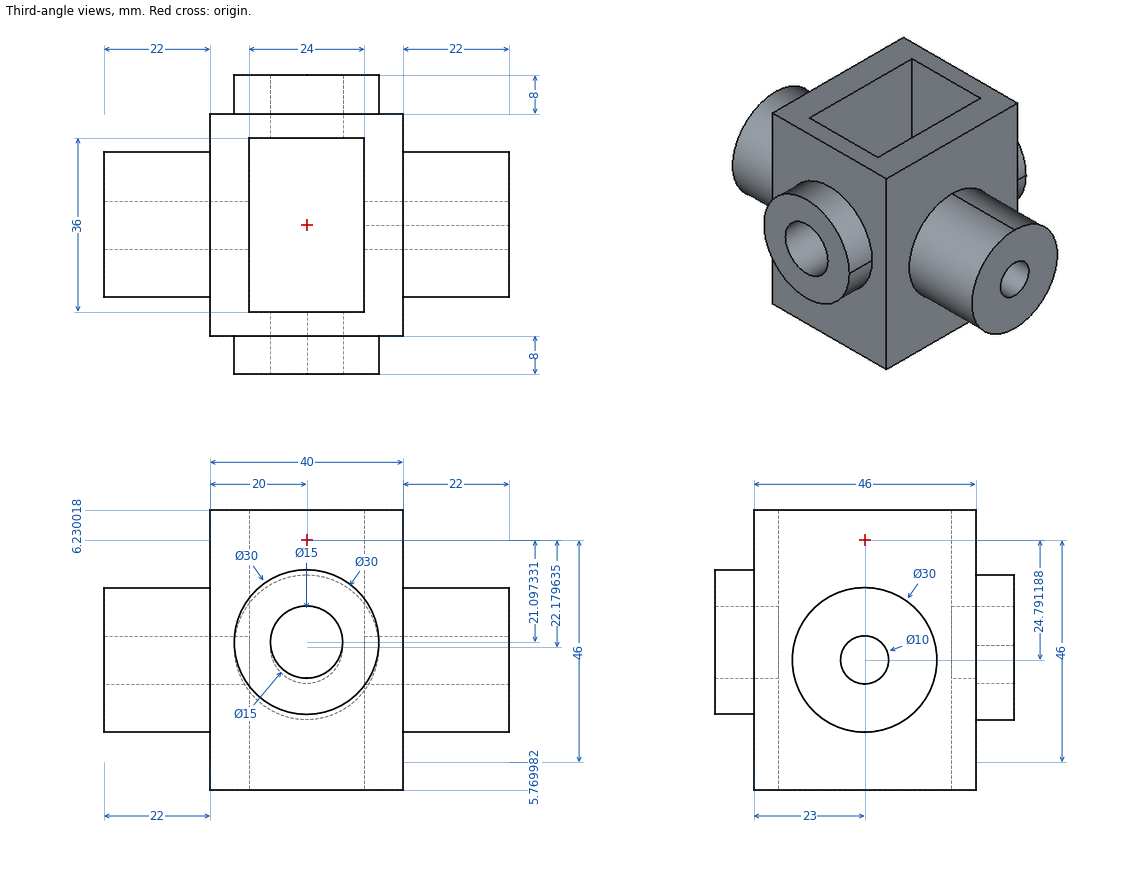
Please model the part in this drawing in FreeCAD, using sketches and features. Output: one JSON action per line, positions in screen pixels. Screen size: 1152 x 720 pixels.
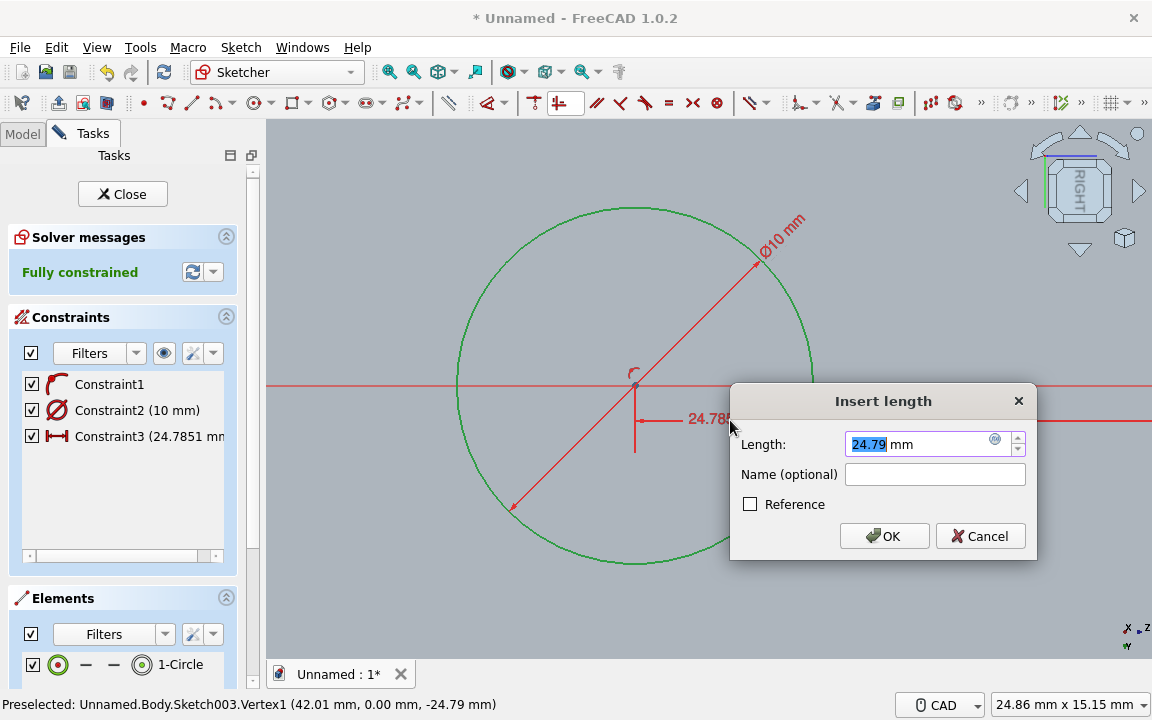
{"action": "type", "text": "24.791188"}
{"action": "key", "text": "Return"}
{"action": "key", "text": "Escape"}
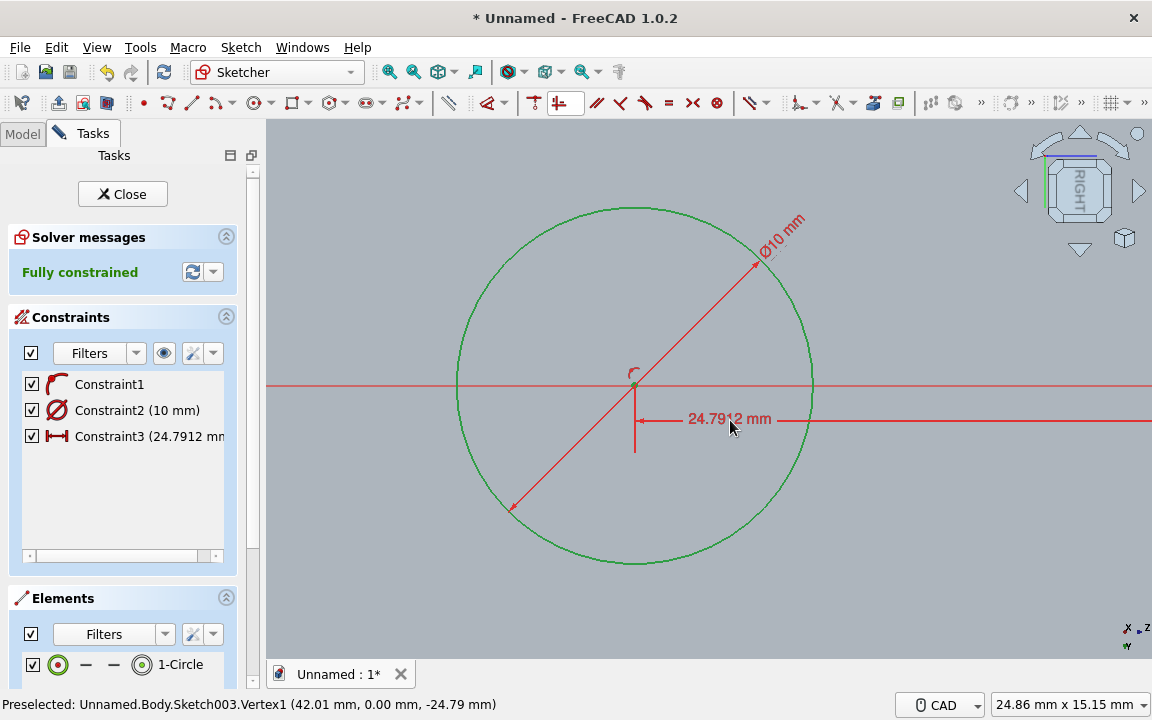
{"action": "left_click", "coordinate": [123, 194]}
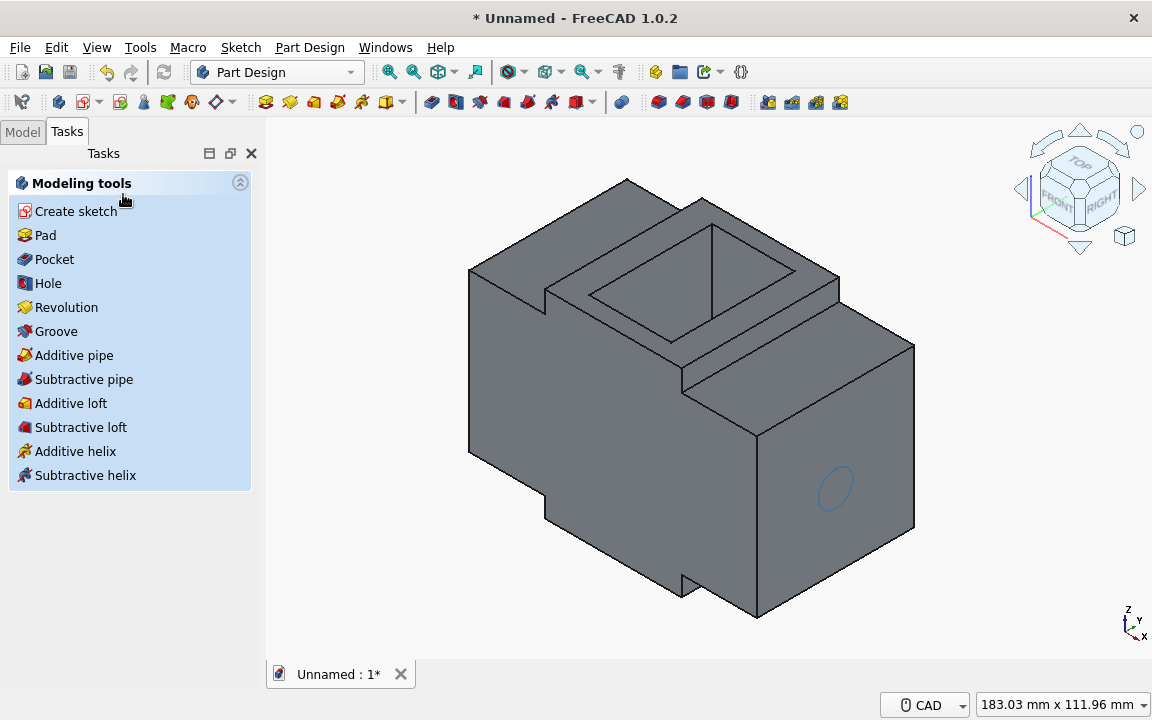
{"action": "left_click", "coordinate": [432, 102]}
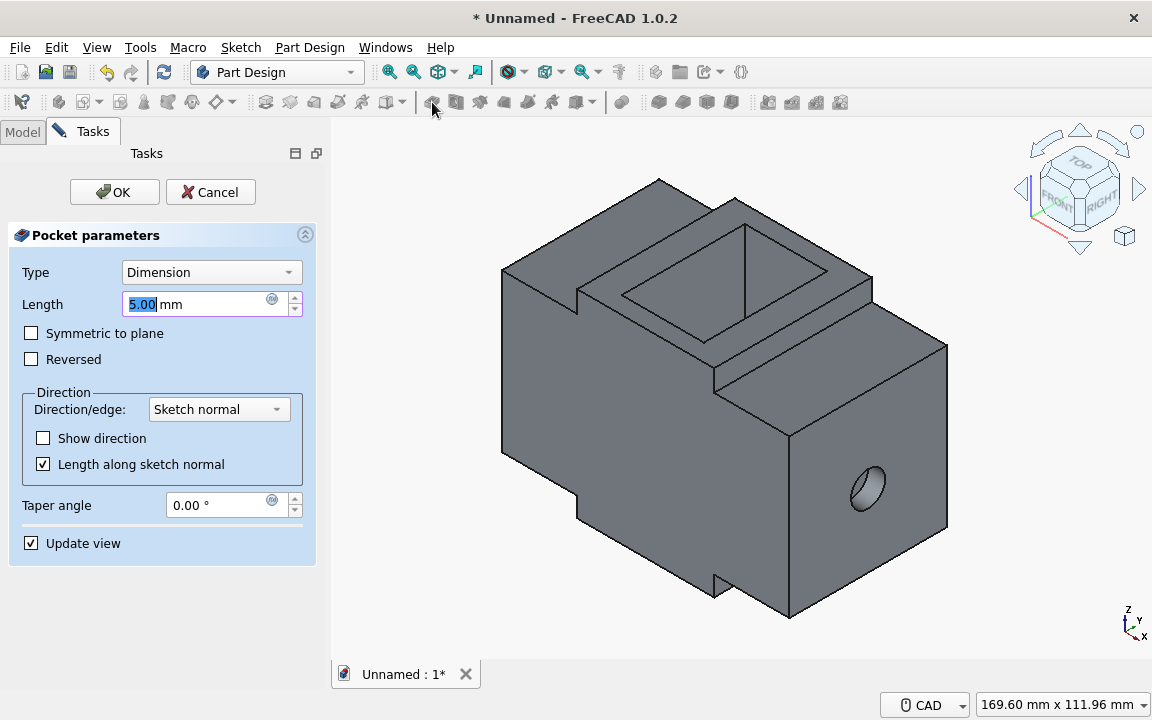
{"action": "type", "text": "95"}
{"action": "key", "text": "Tab"}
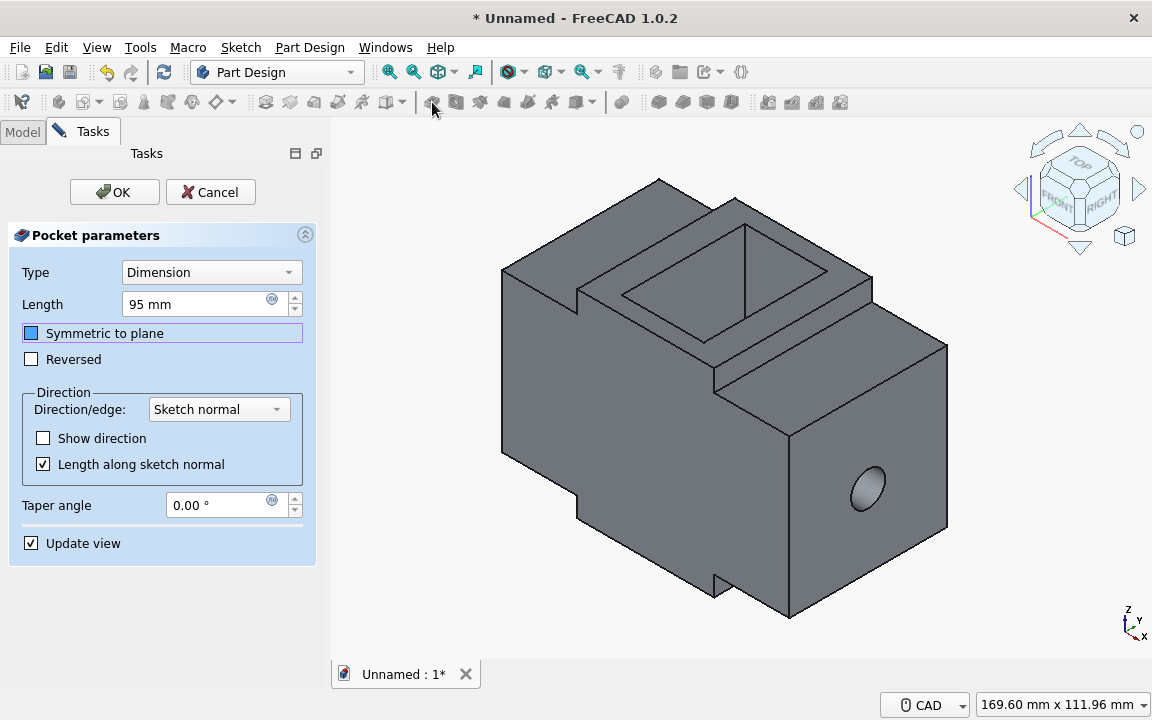
{"action": "left_click", "coordinate": [115, 192]}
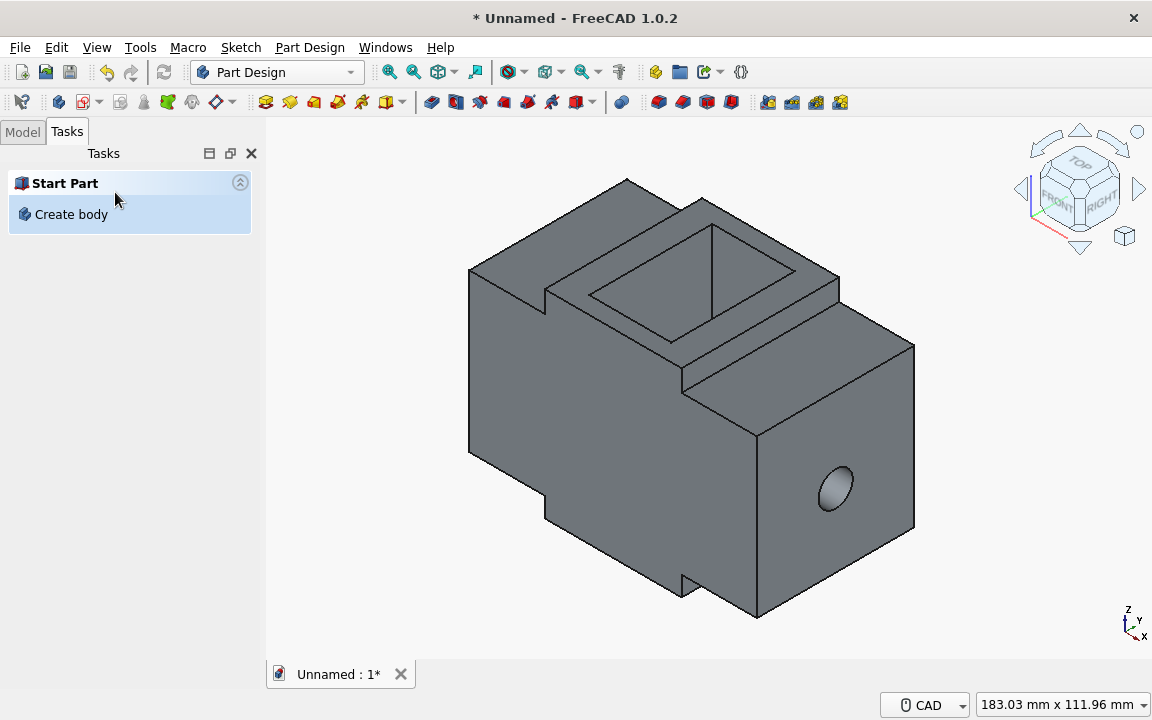
{"action": "left_click", "coordinate": [791, 481]}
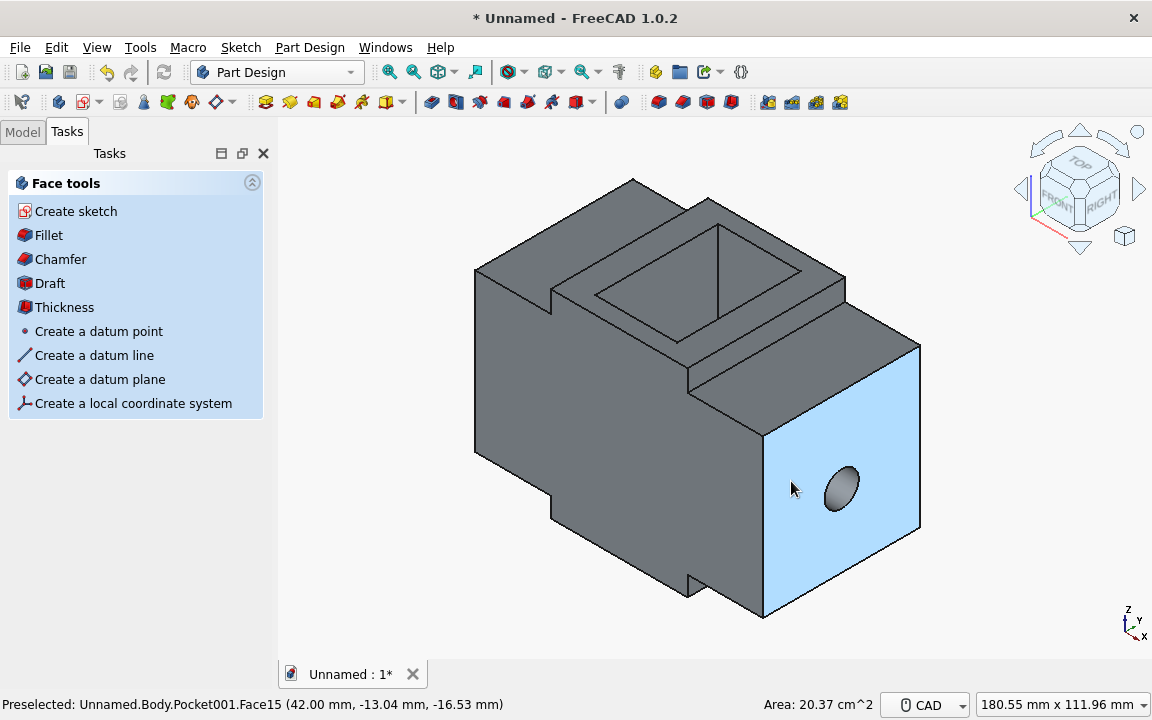
{"action": "left_click", "coordinate": [84, 102]}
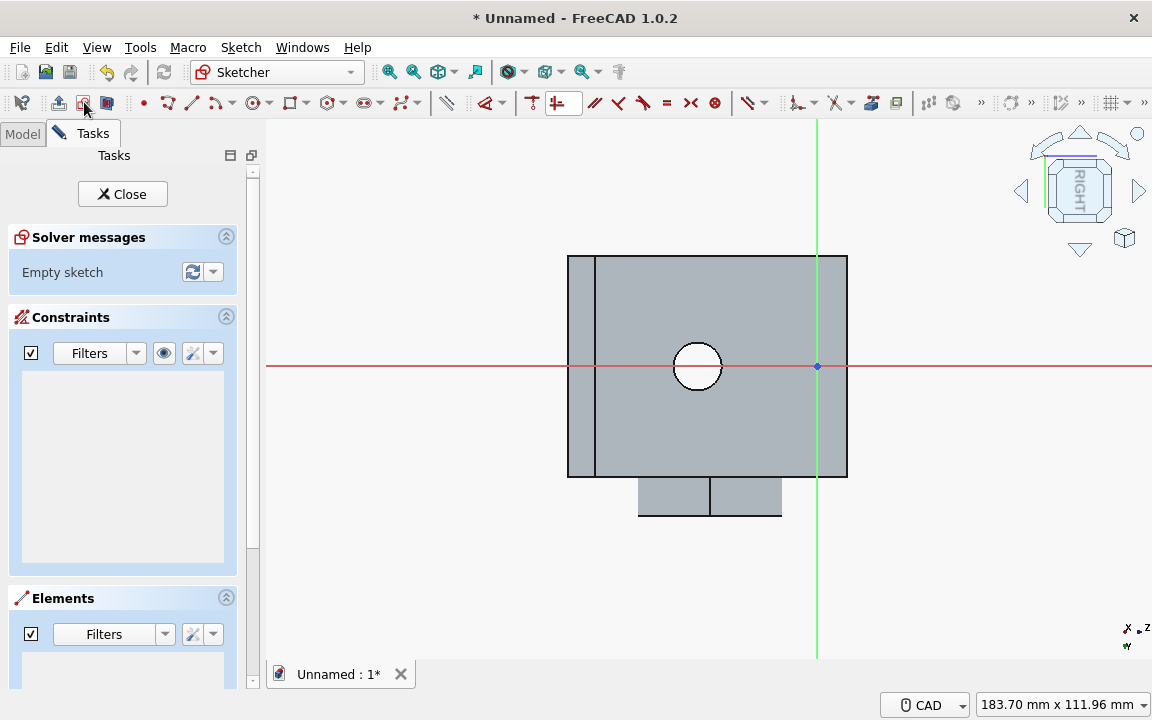
{"action": "scroll", "coordinate": [840, 321], "scroll_direction": "up", "scroll_amount": 2}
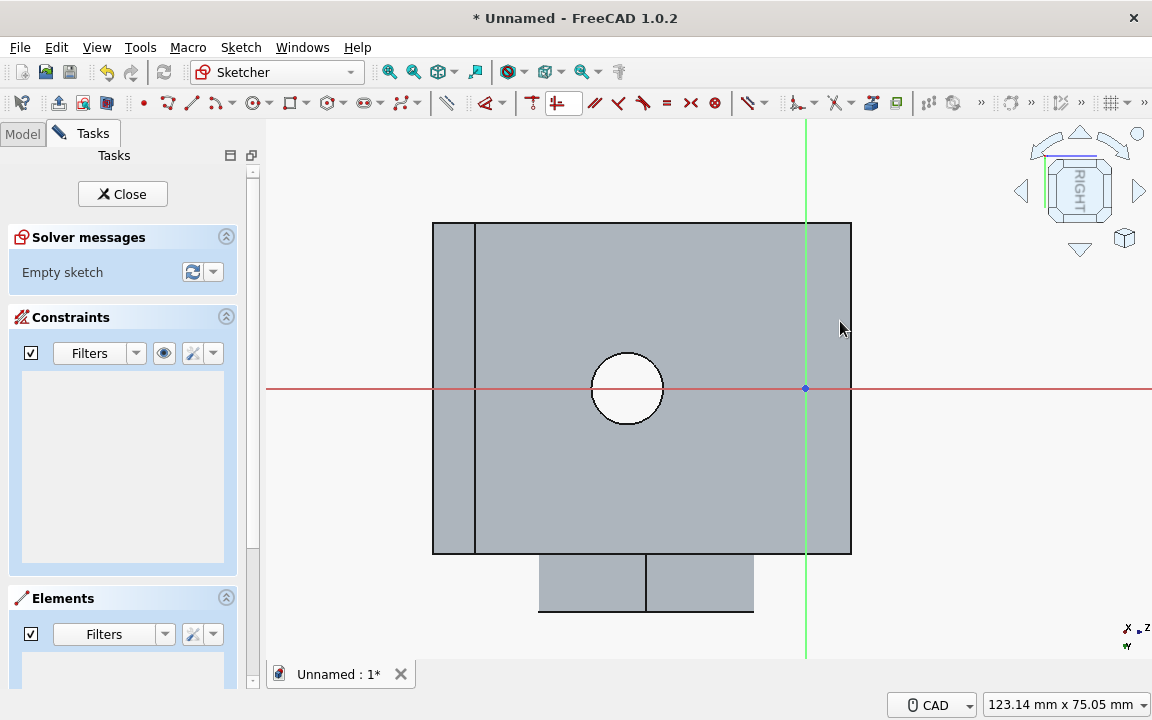
{"action": "left_click", "coordinate": [290, 104]}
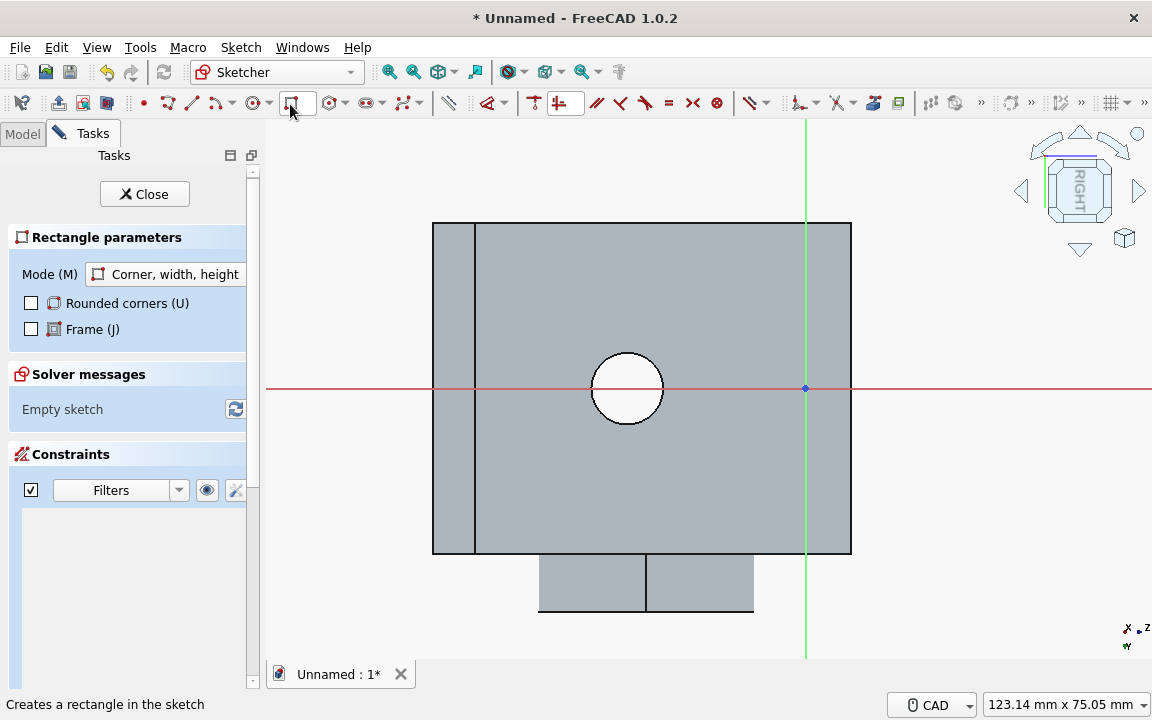
{"action": "left_click", "coordinate": [475, 223]}
{"action": "left_click", "coordinate": [806, 554]}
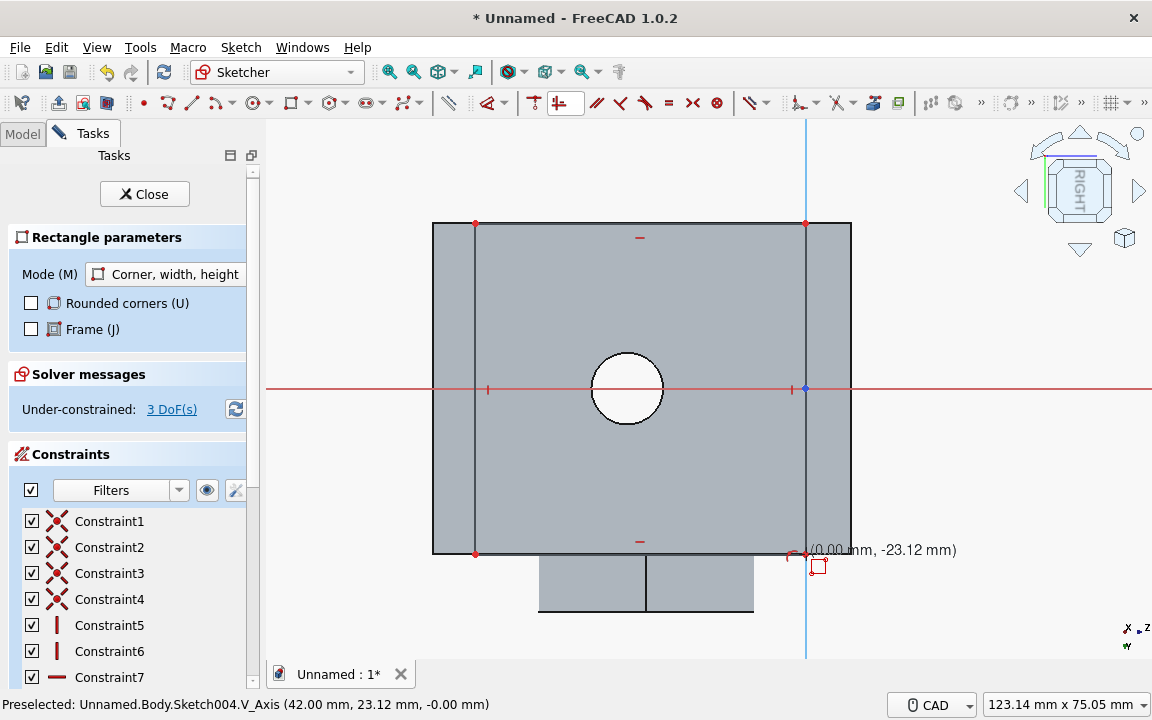
{"action": "left_click", "coordinate": [254, 104]}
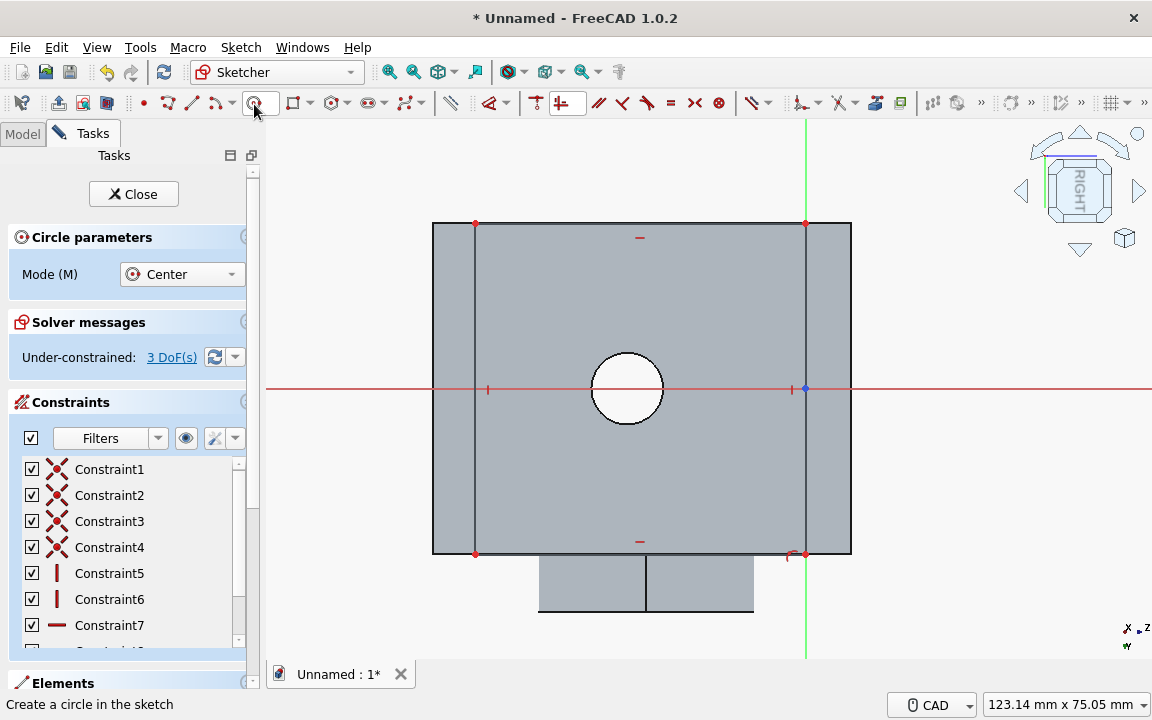
{"action": "left_click", "coordinate": [627, 389]}
{"action": "left_click", "coordinate": [653, 363]}